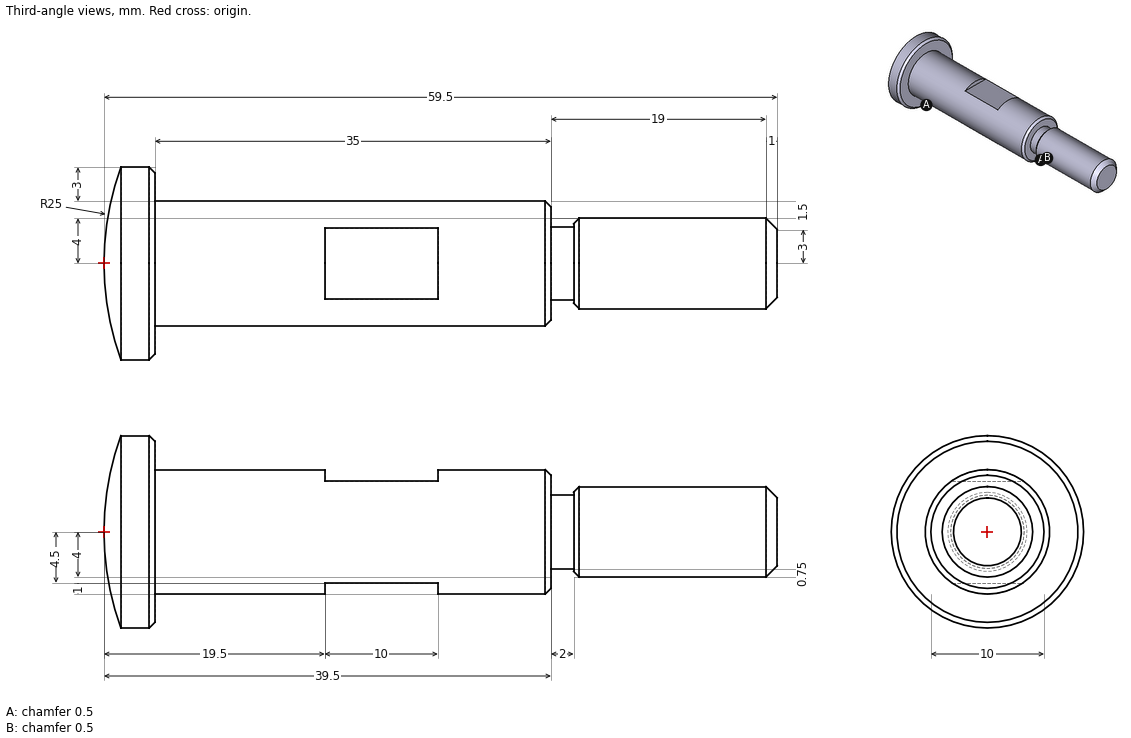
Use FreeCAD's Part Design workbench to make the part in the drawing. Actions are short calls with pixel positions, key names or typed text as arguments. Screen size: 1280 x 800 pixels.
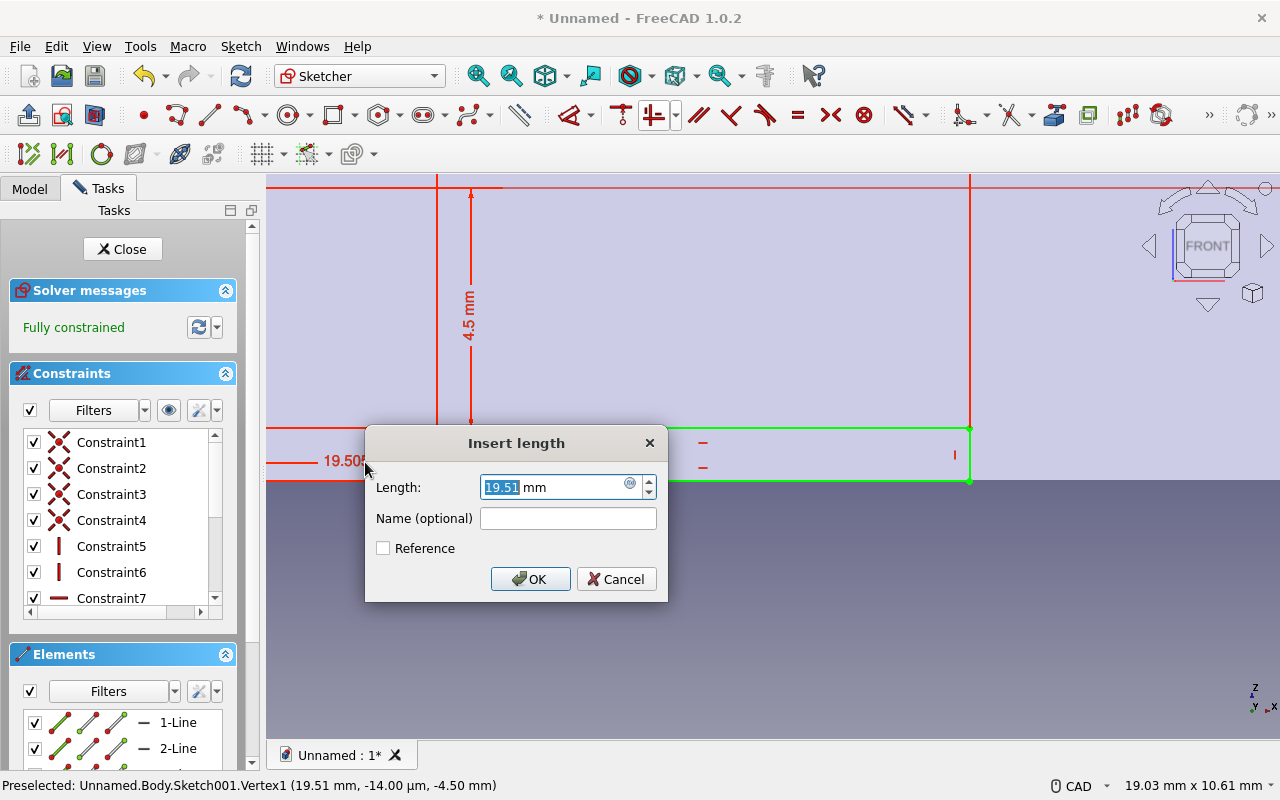
text(19.5)
key(Return)
key(Escape)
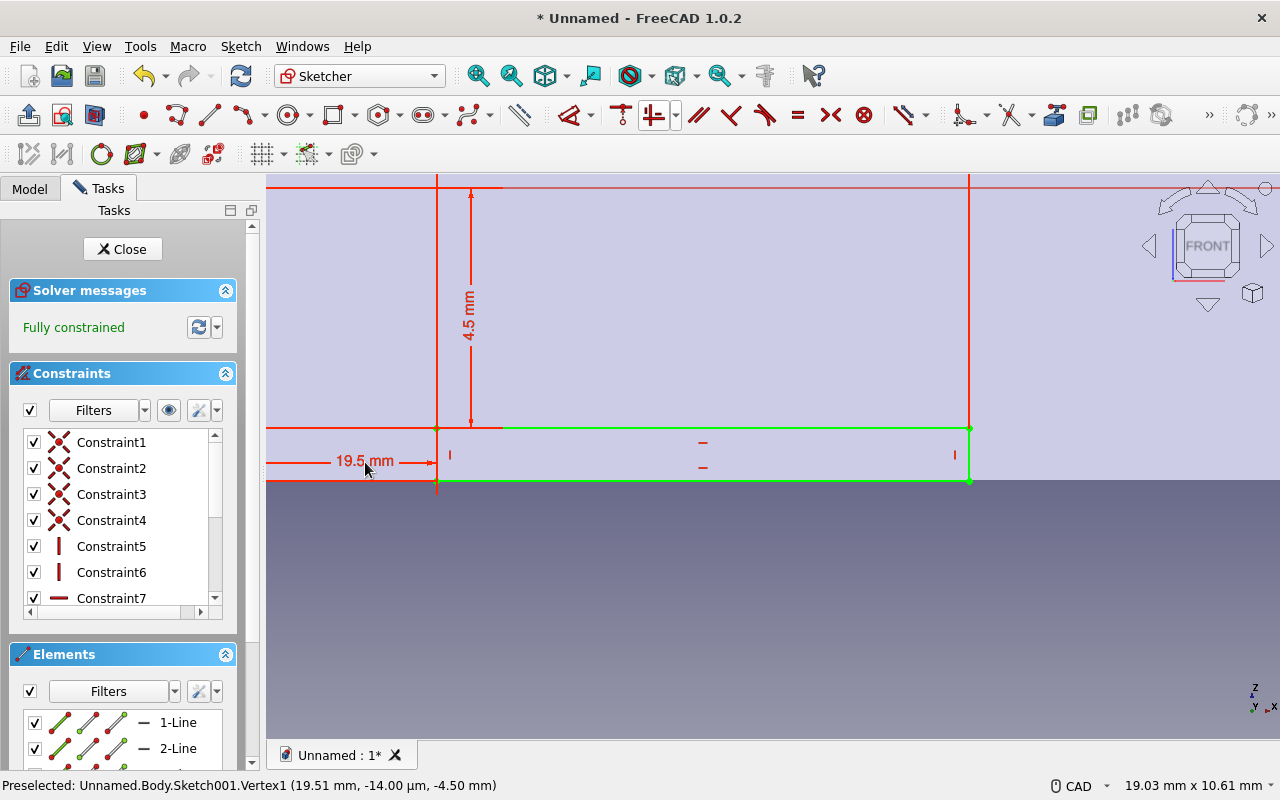
click(123, 249)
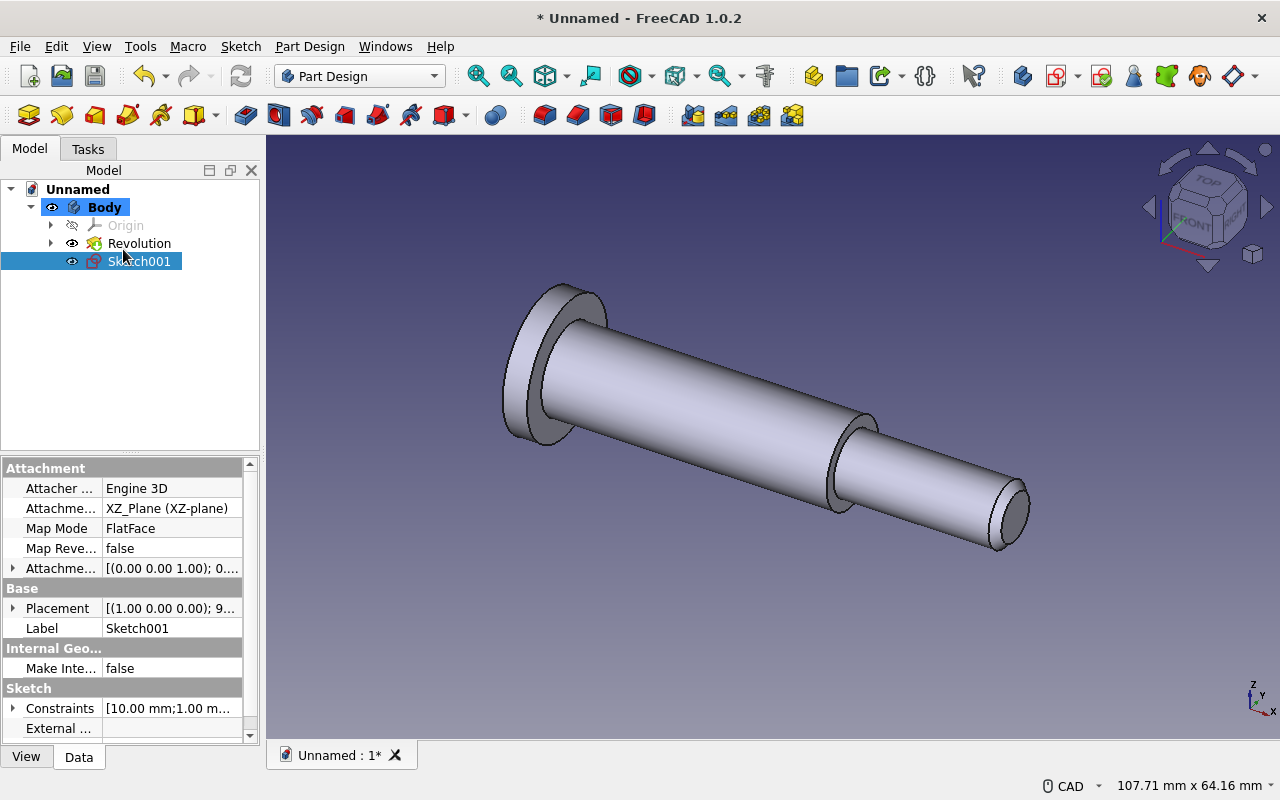
click(246, 116)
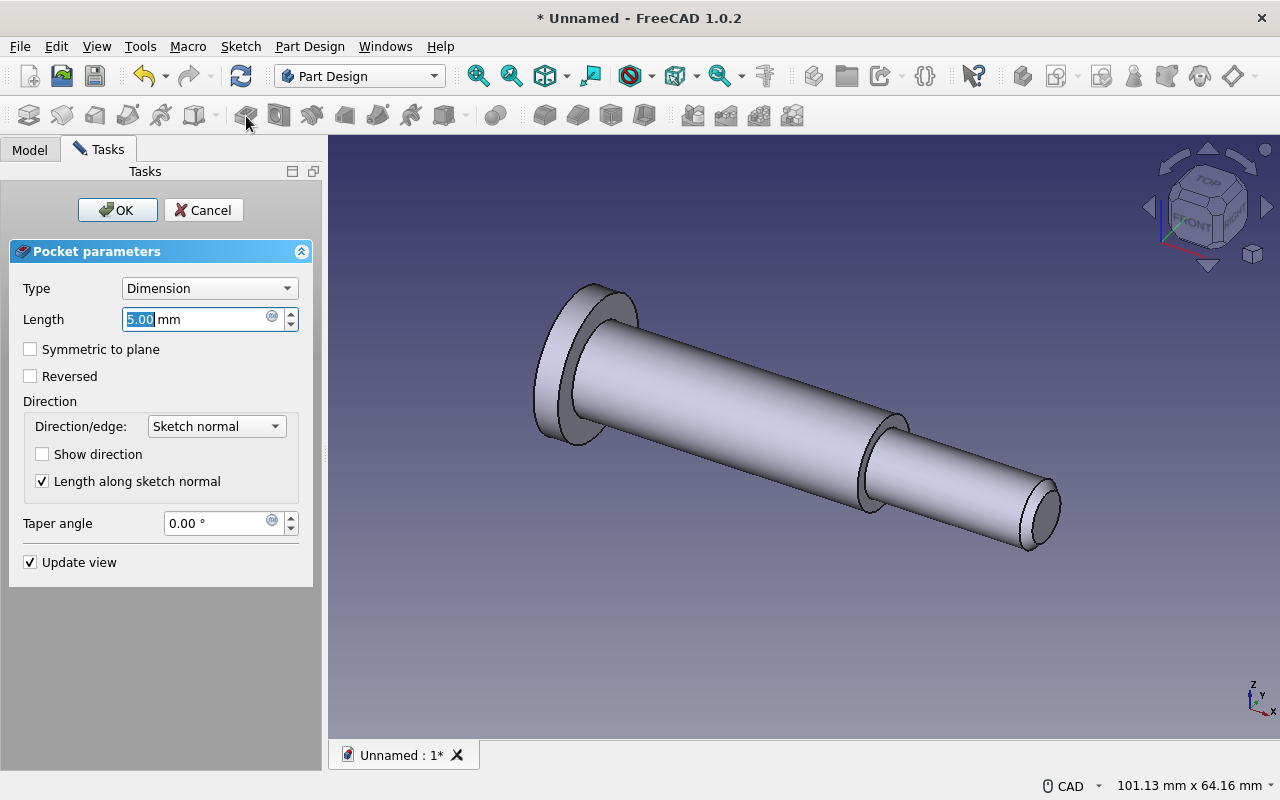
text(10)
key(Tab)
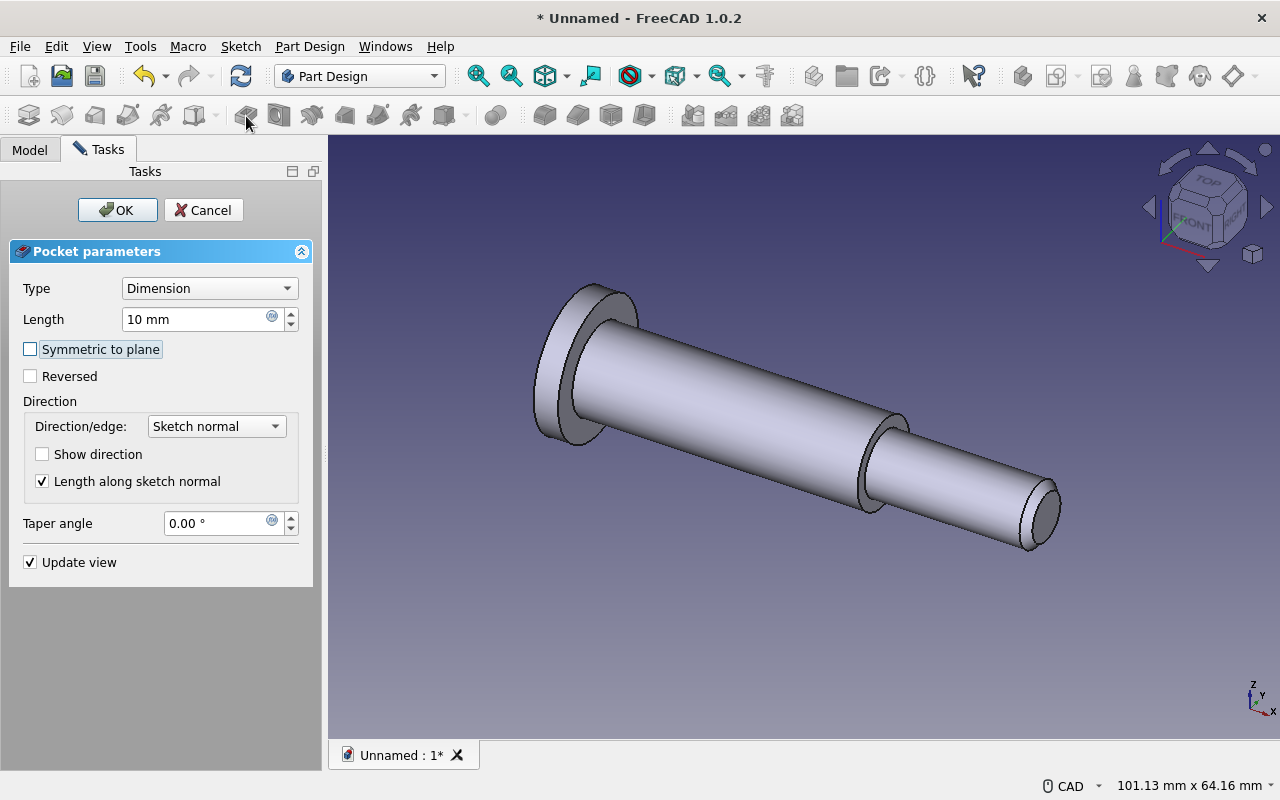
click(31, 349)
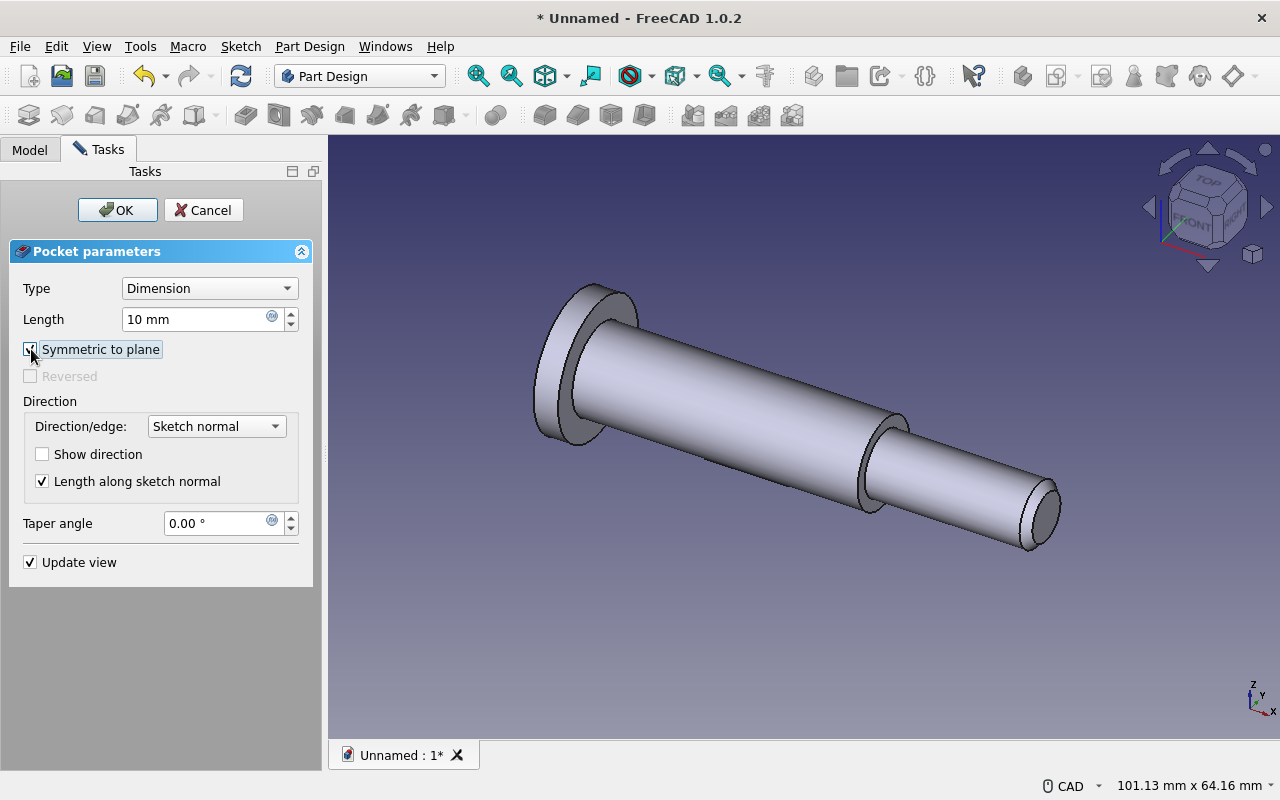
click(118, 210)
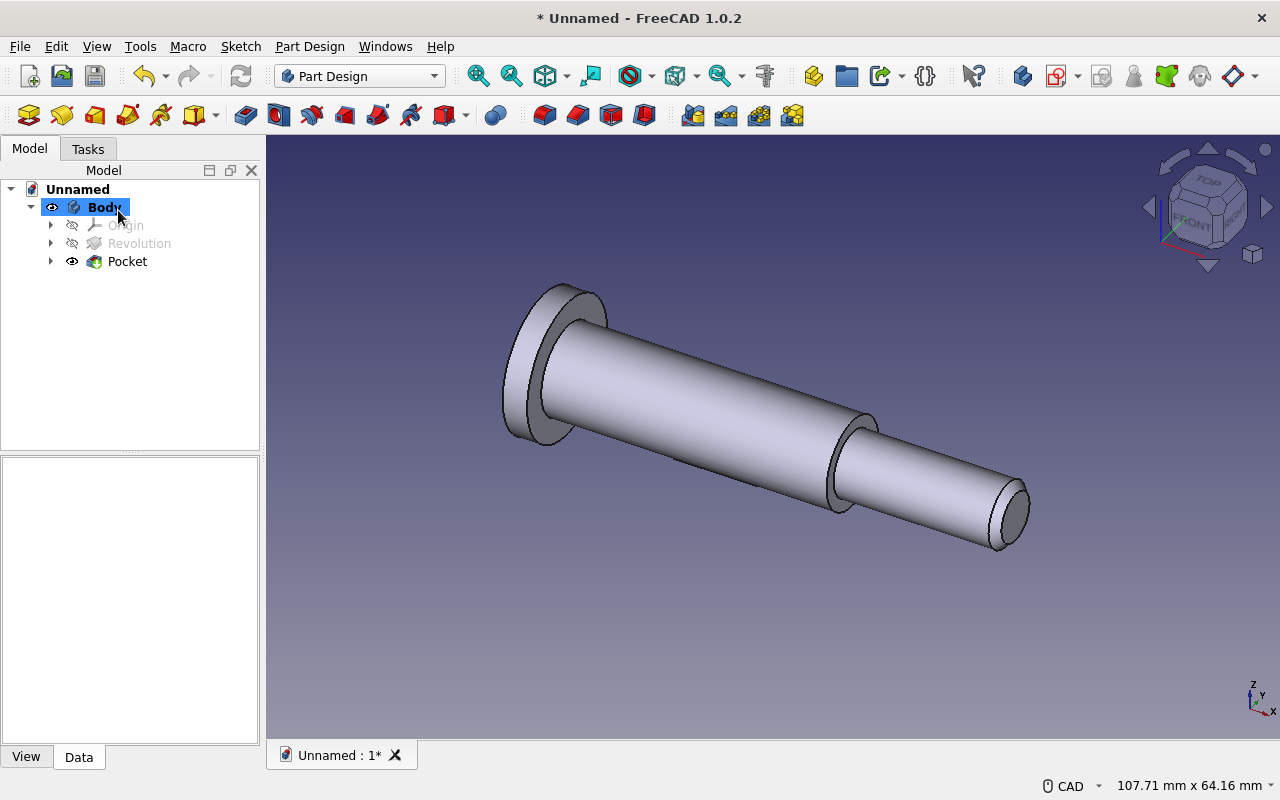
click(117, 261)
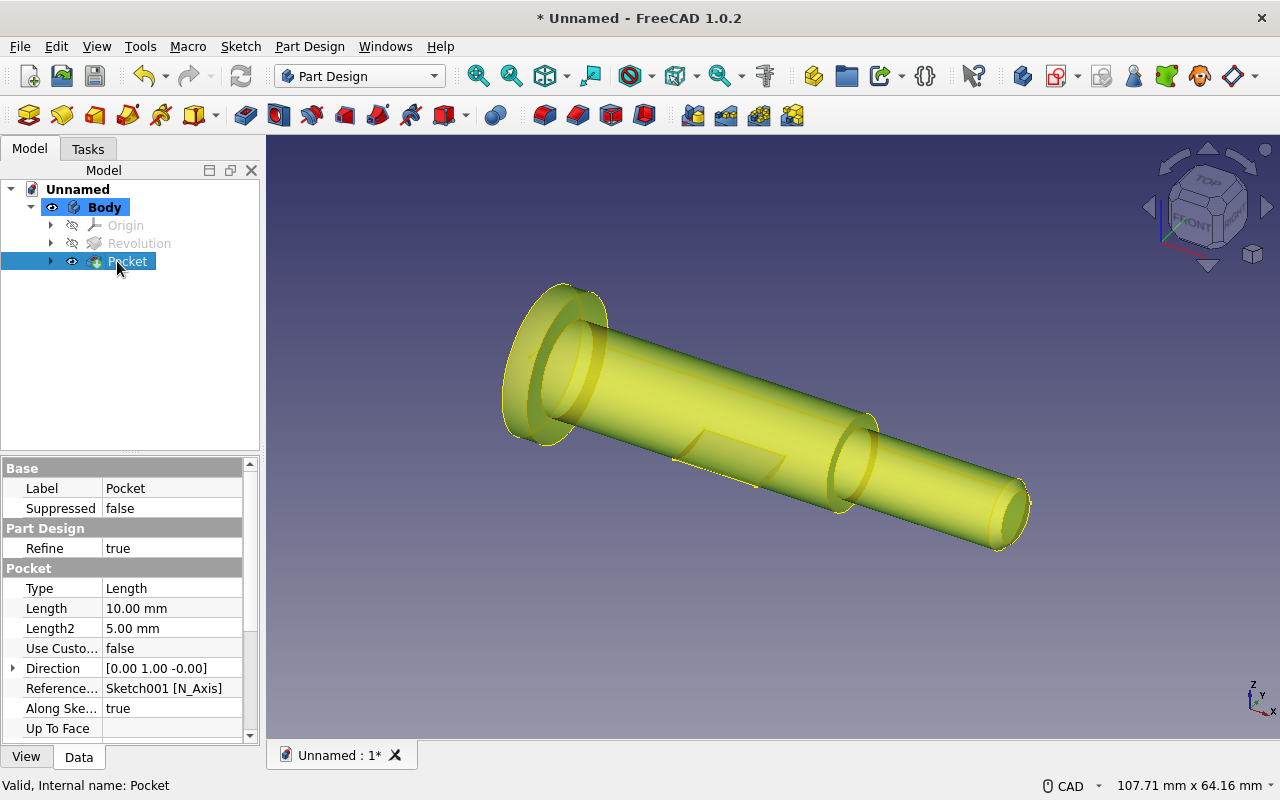
click(693, 116)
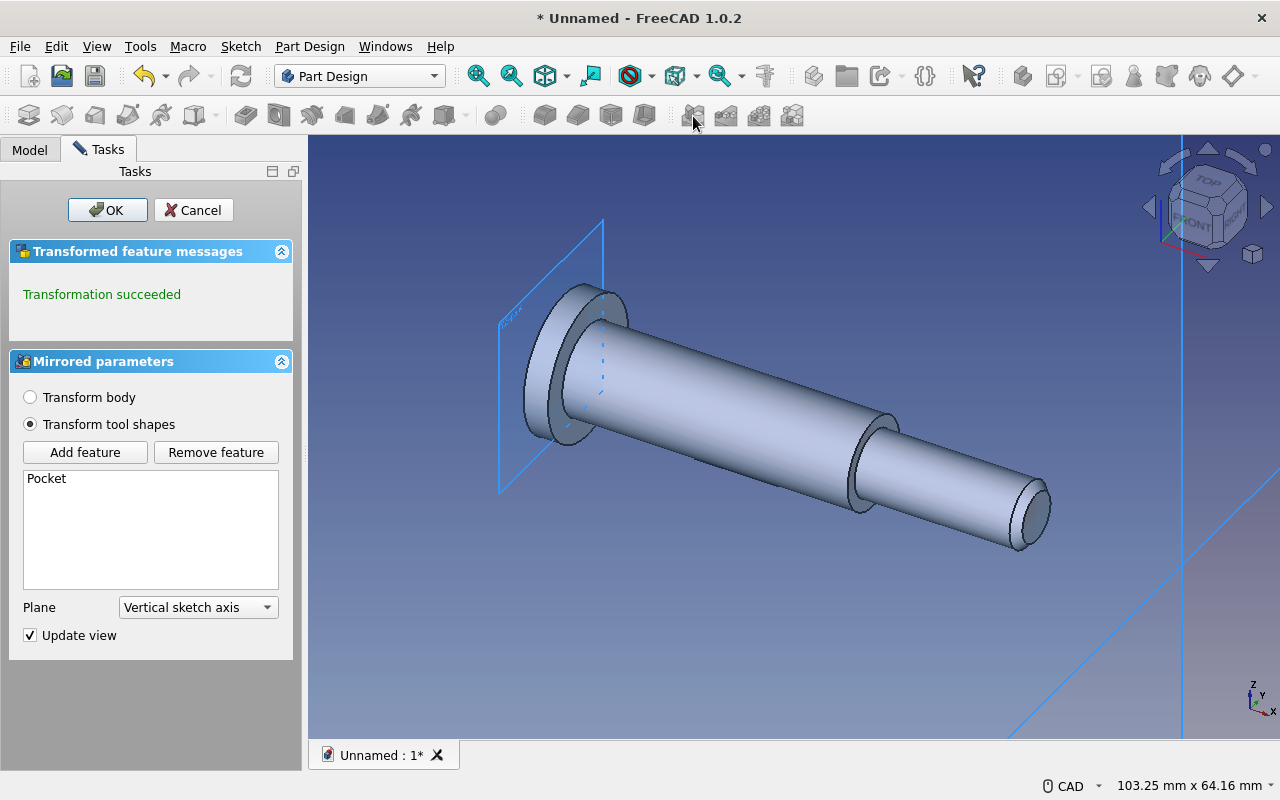
click(199, 608)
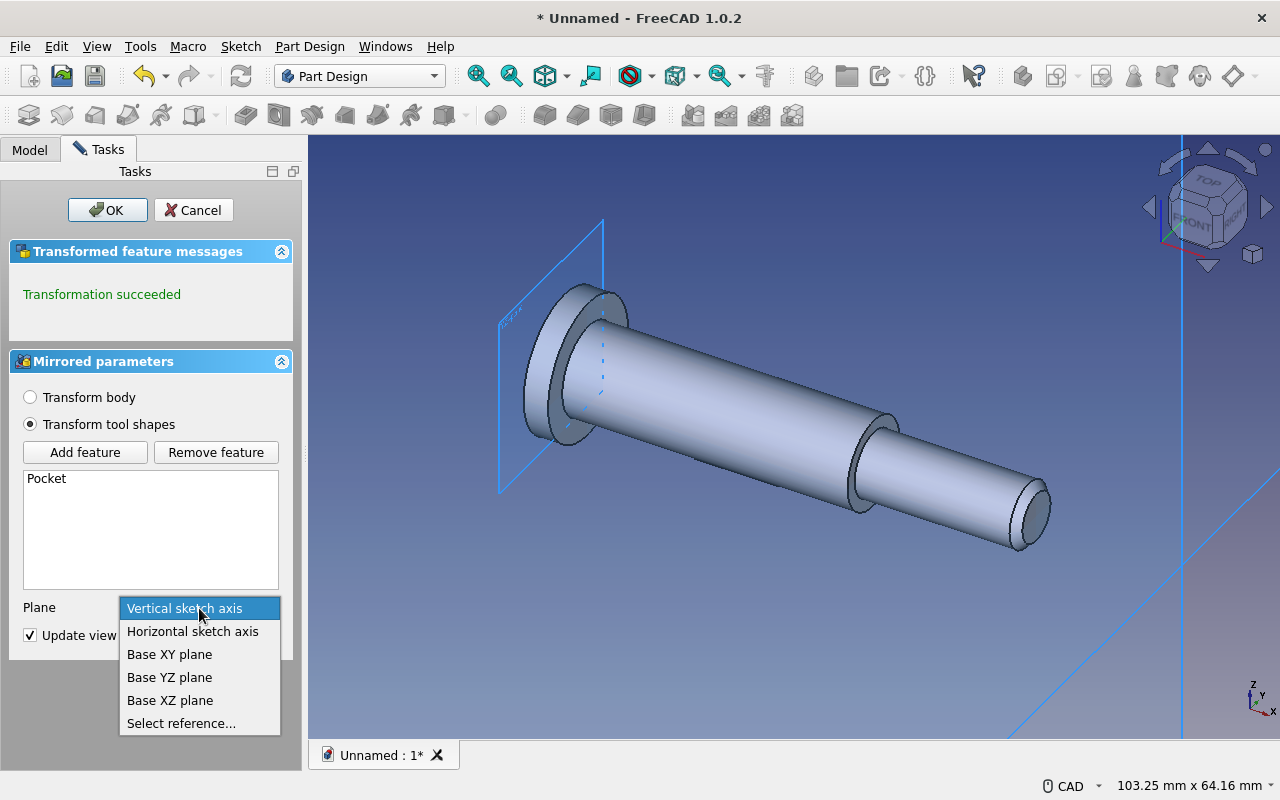
click(198, 654)